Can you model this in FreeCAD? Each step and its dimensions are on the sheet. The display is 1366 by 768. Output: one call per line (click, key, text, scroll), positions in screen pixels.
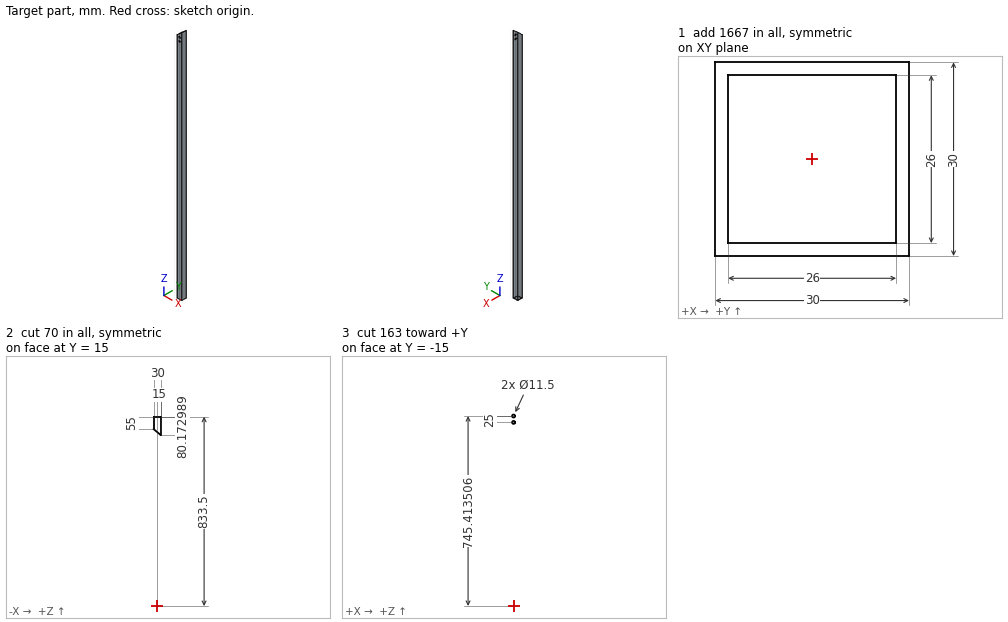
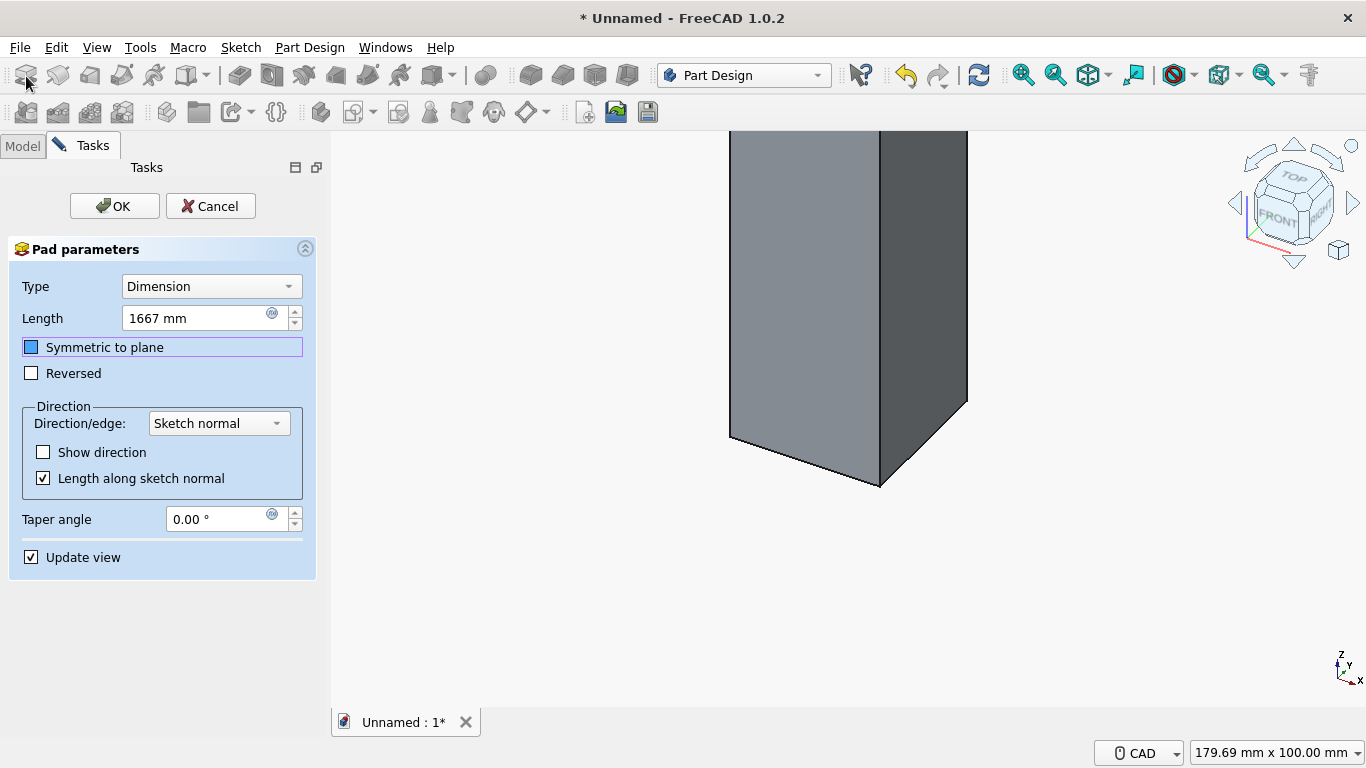
click(30, 347)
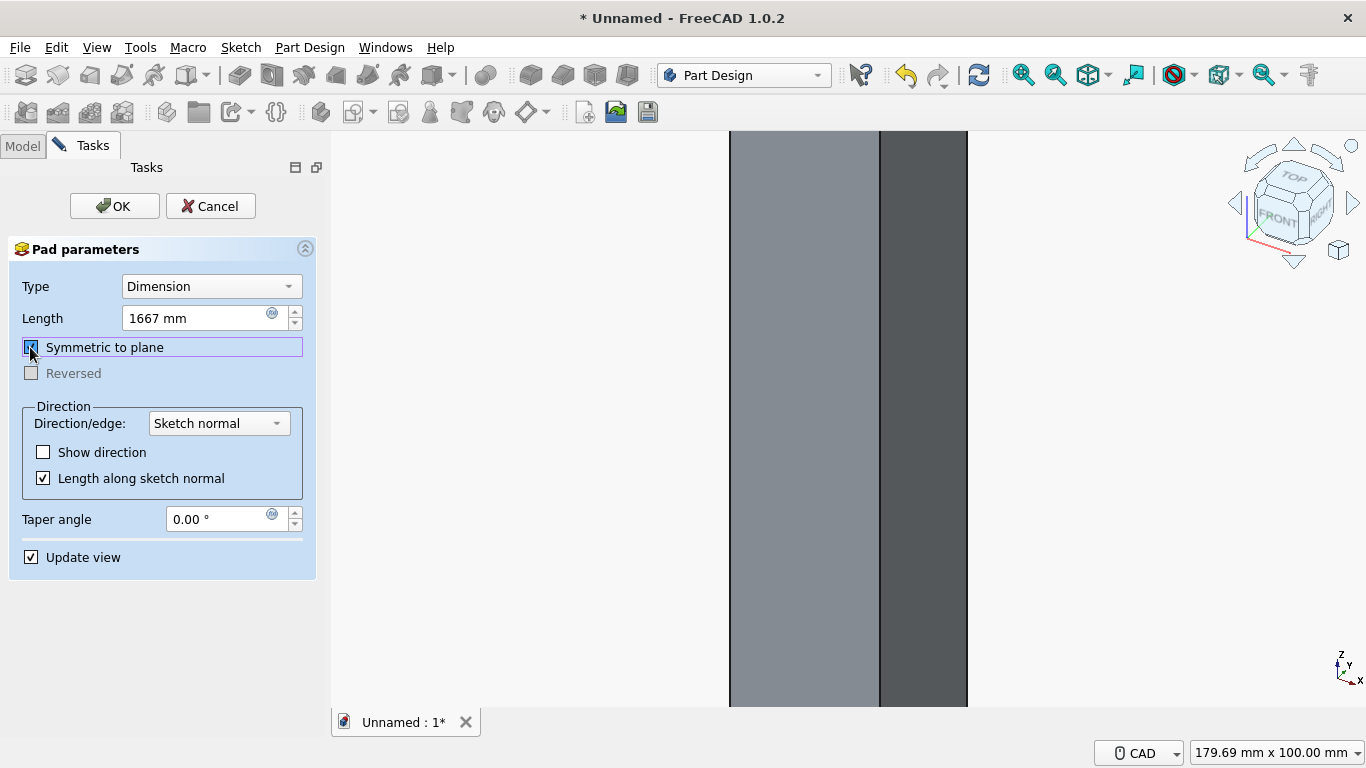
click(115, 206)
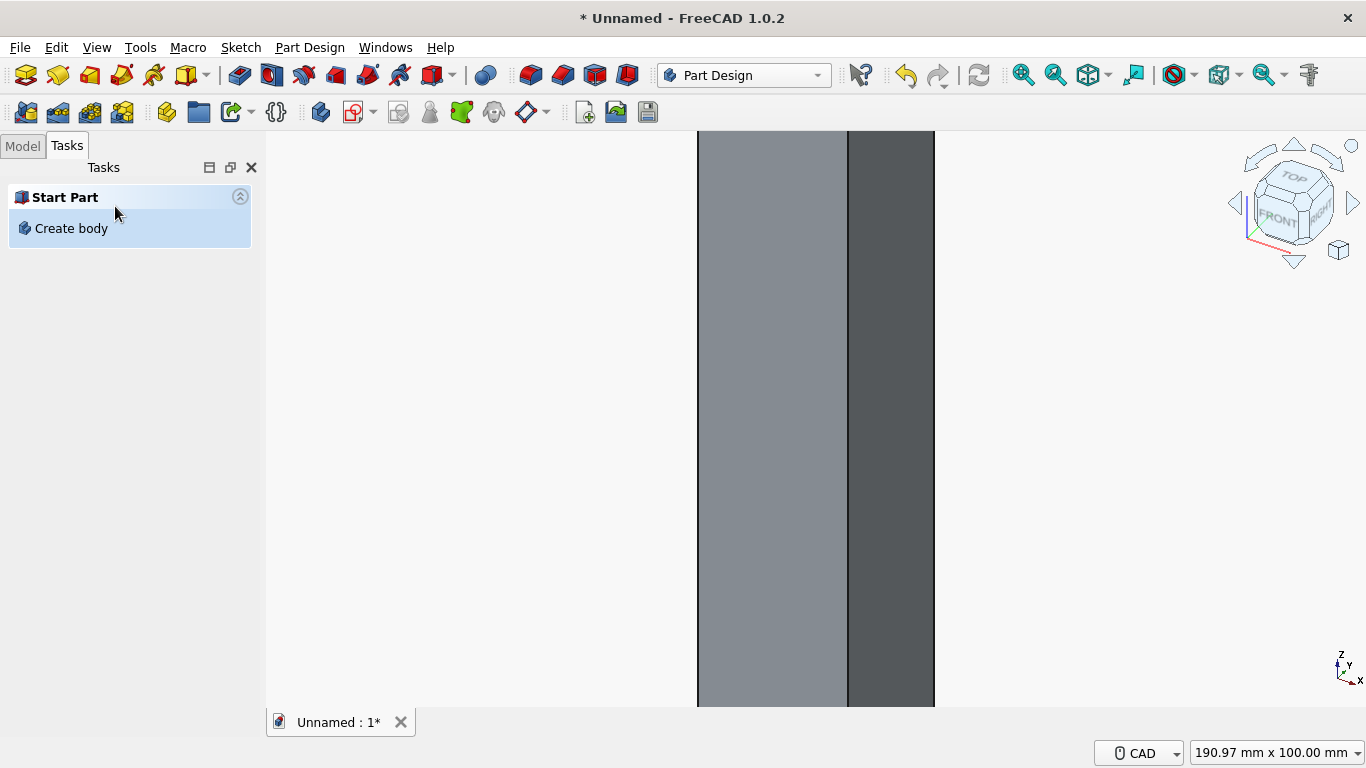
click(1024, 76)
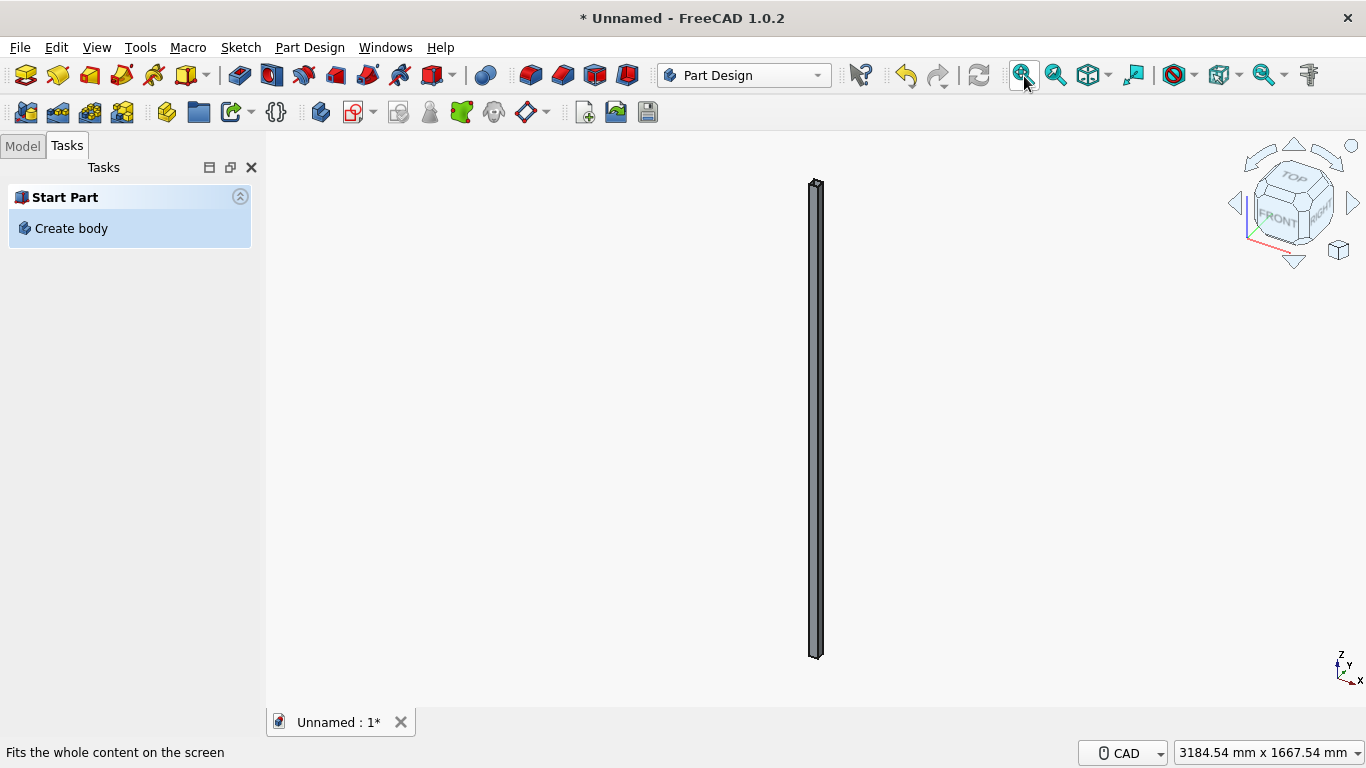
key(4)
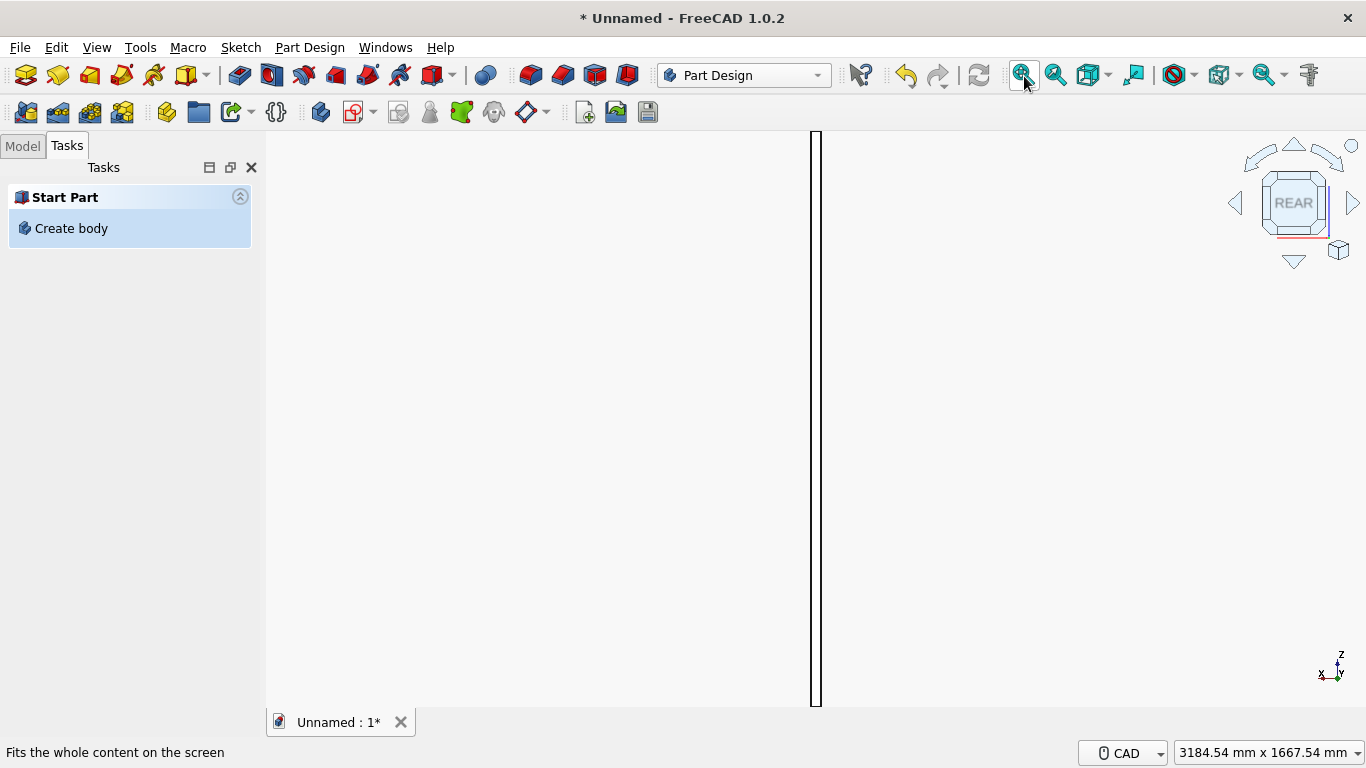
key(v)
key(f)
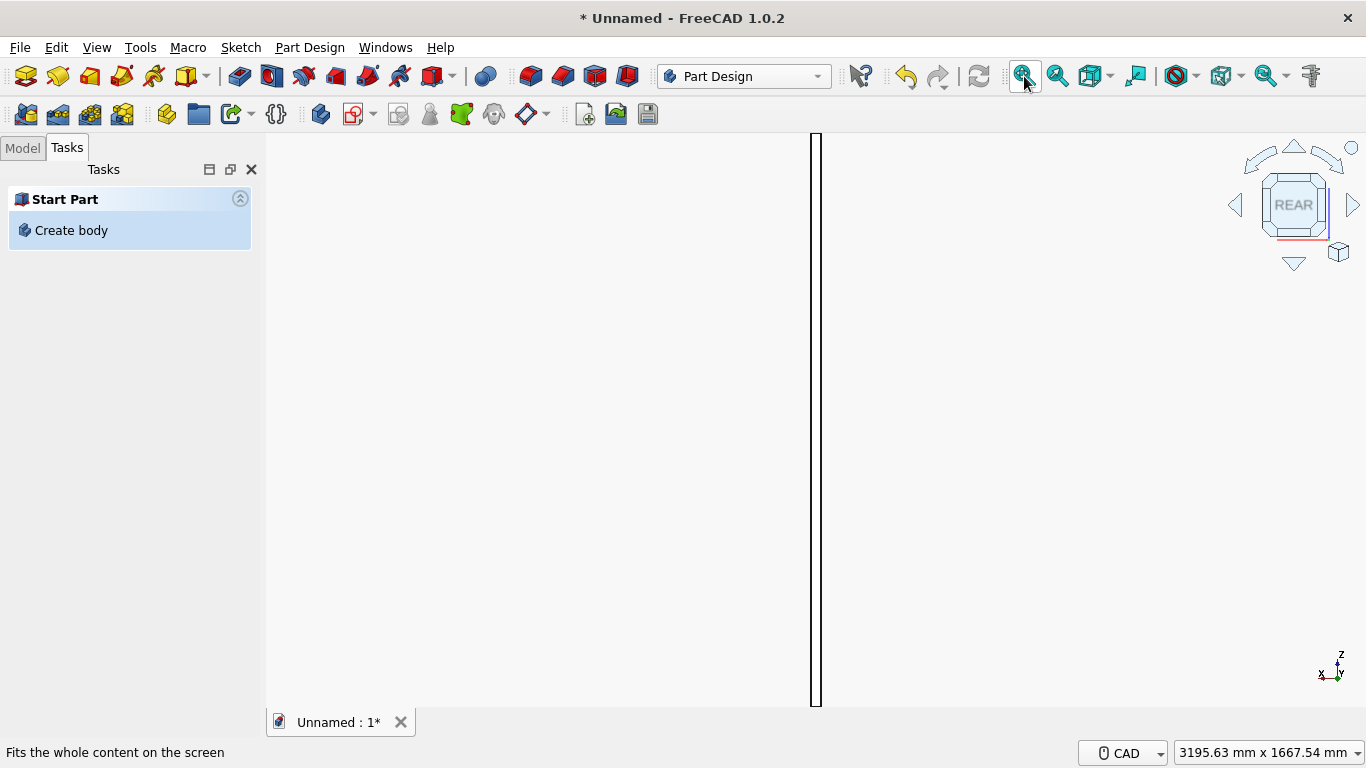
scroll(816, 173, up, 5)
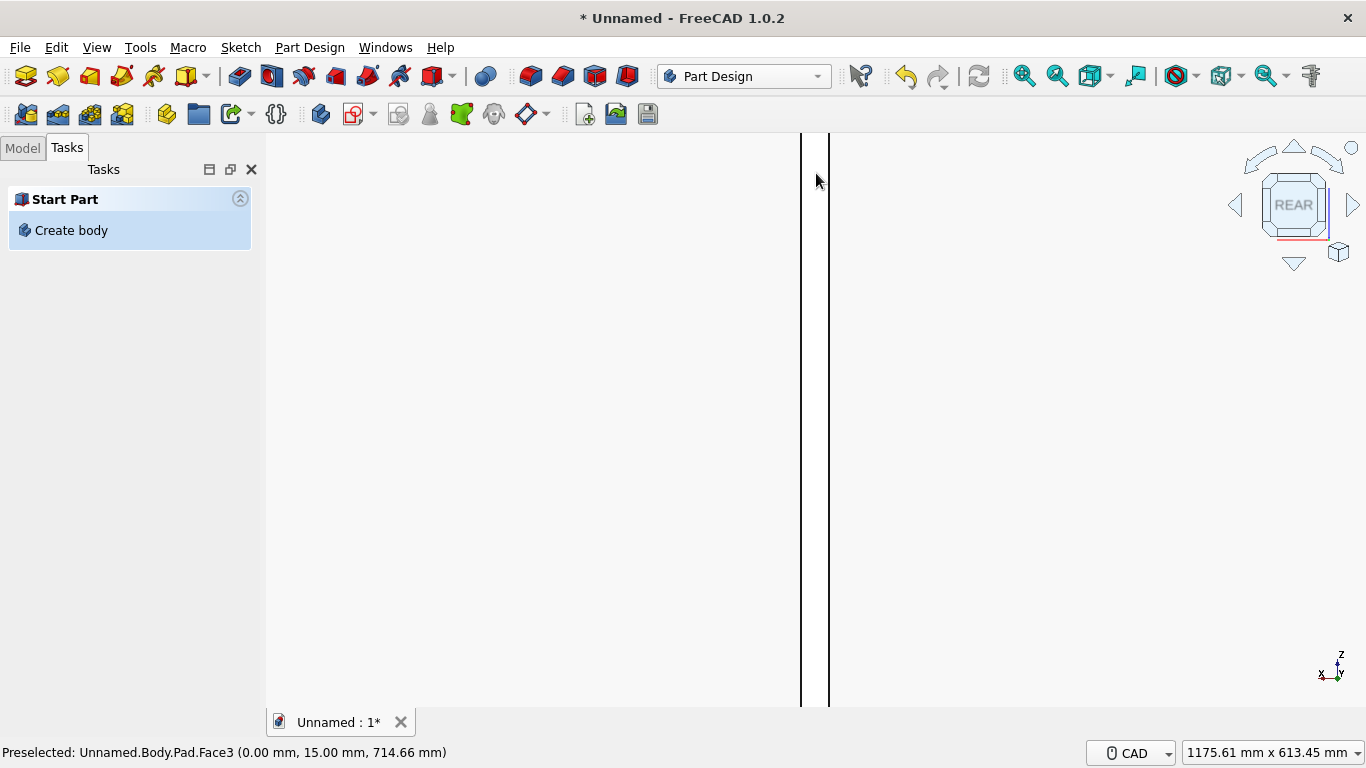
click(815, 175)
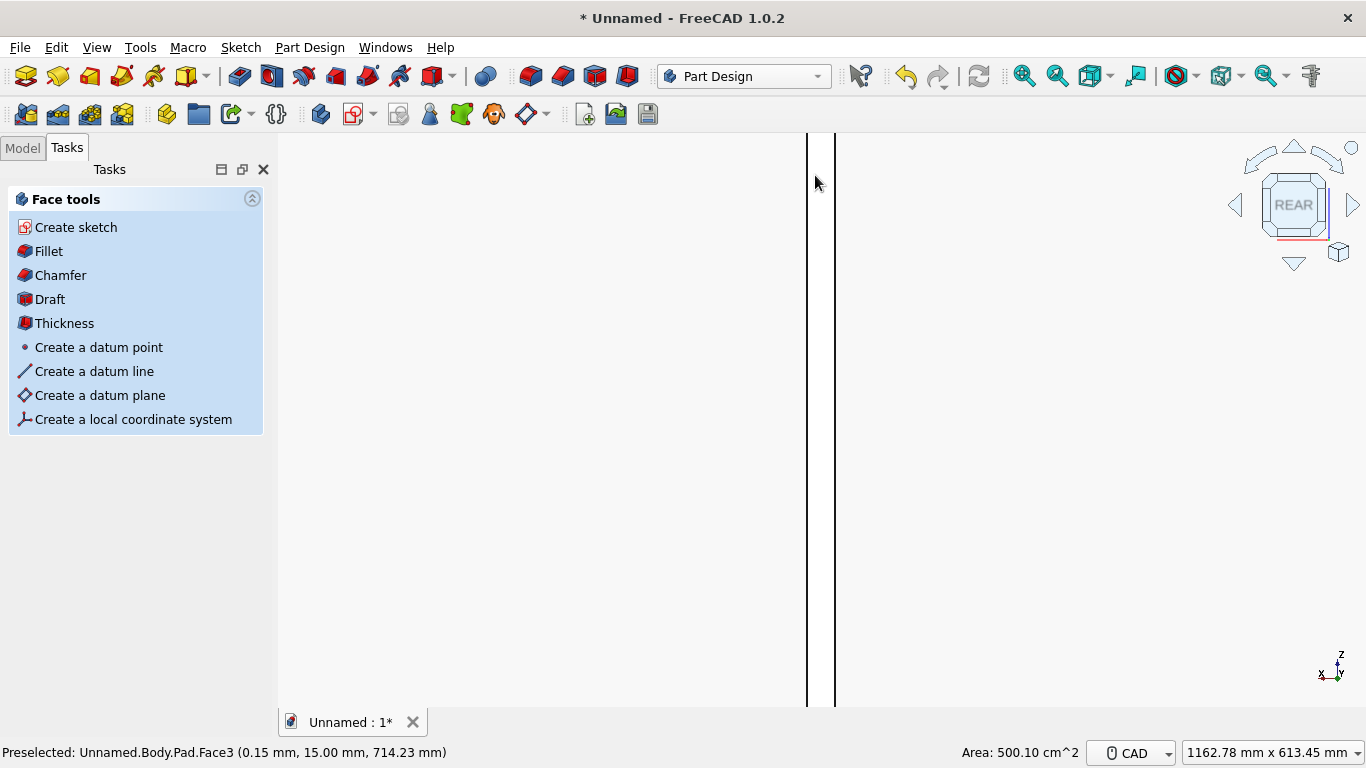
click(354, 114)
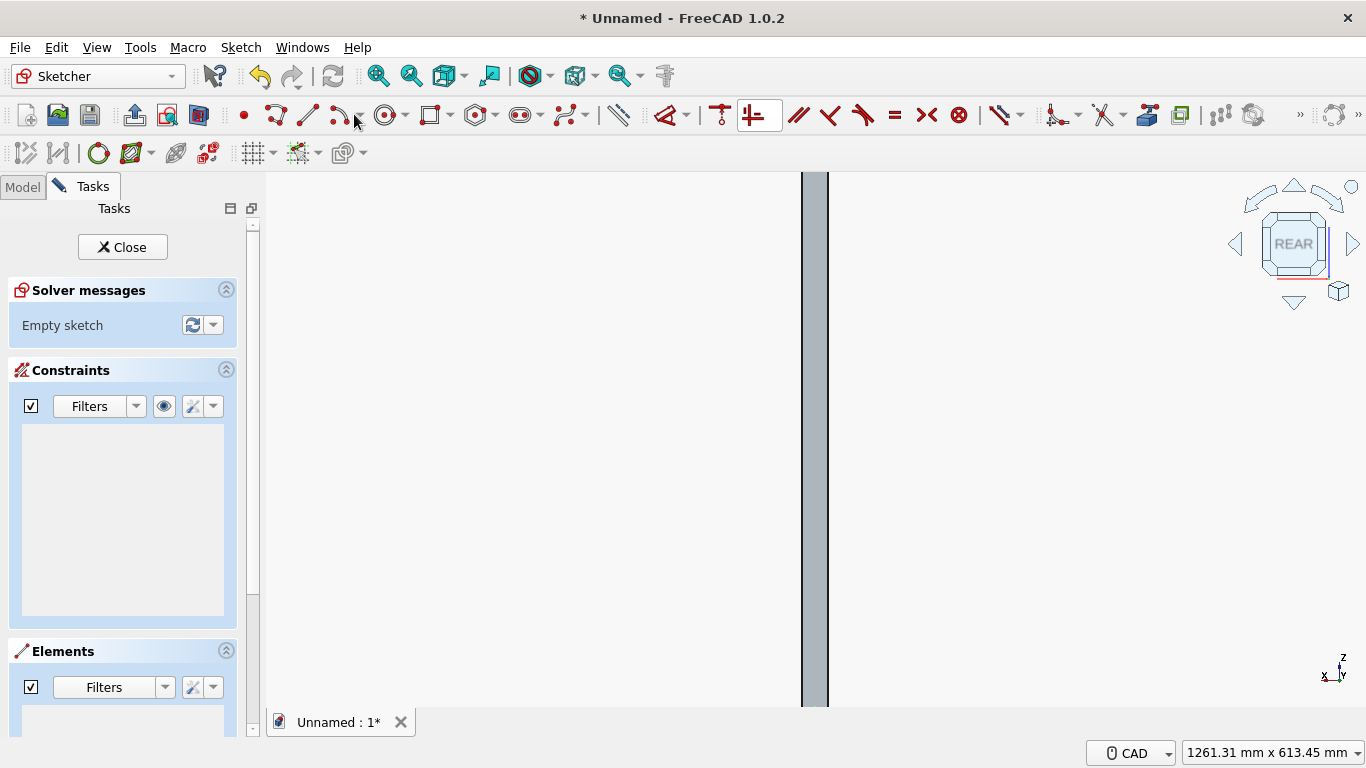
scroll(748, 440, down, 5)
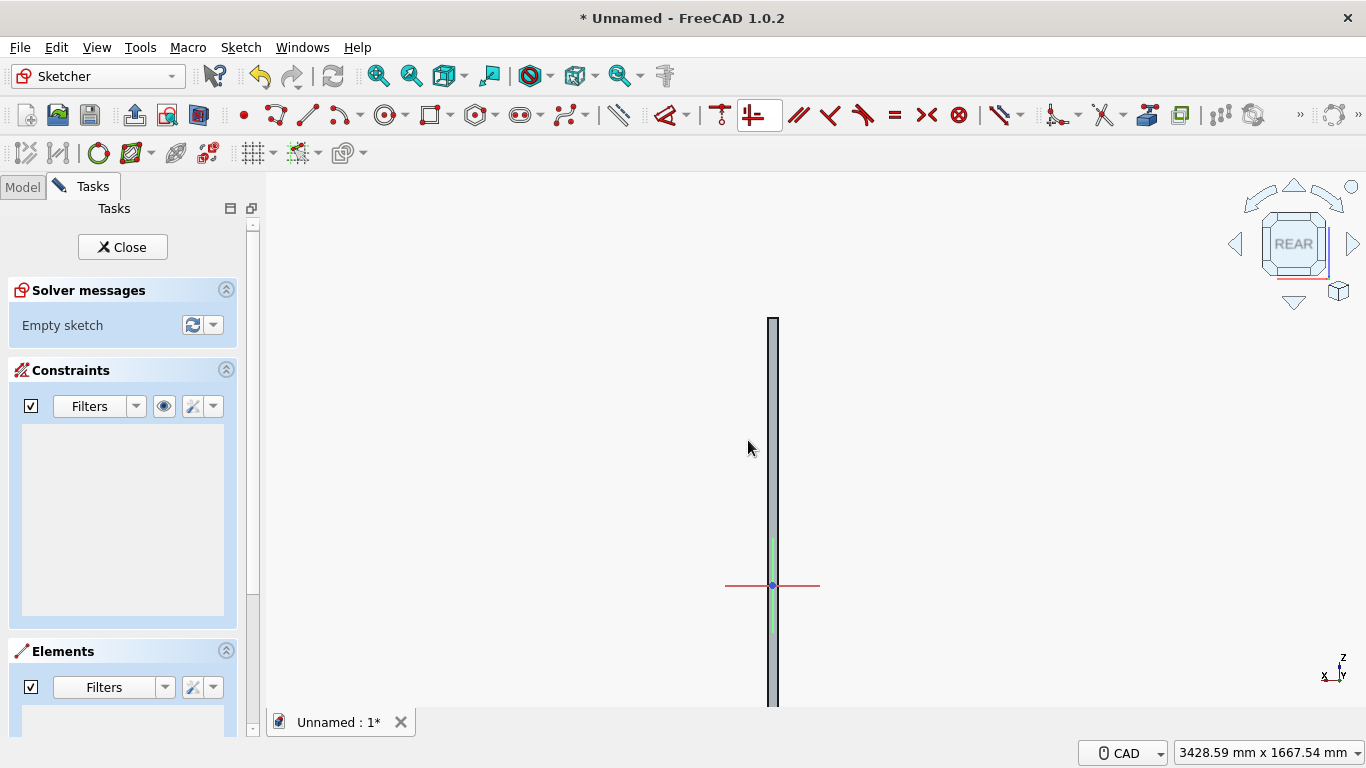
scroll(775, 322, up, 13)